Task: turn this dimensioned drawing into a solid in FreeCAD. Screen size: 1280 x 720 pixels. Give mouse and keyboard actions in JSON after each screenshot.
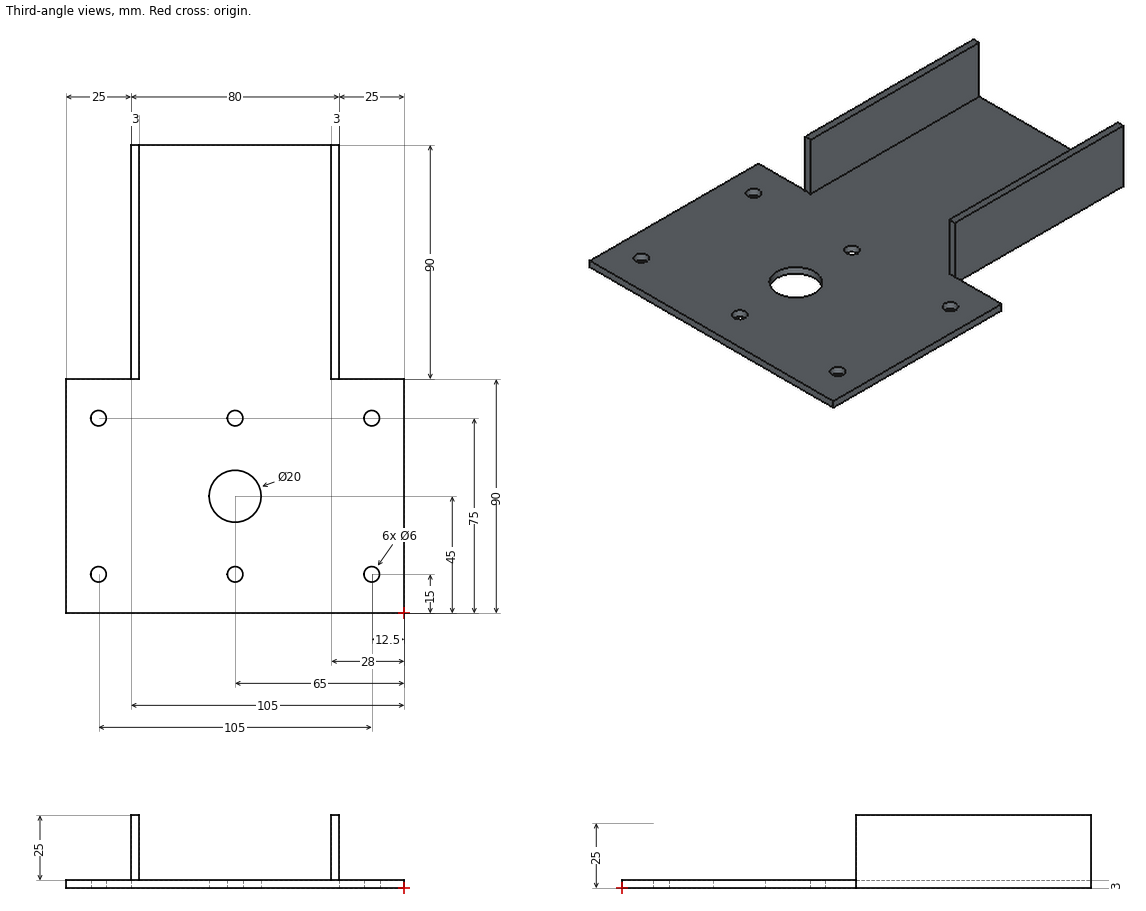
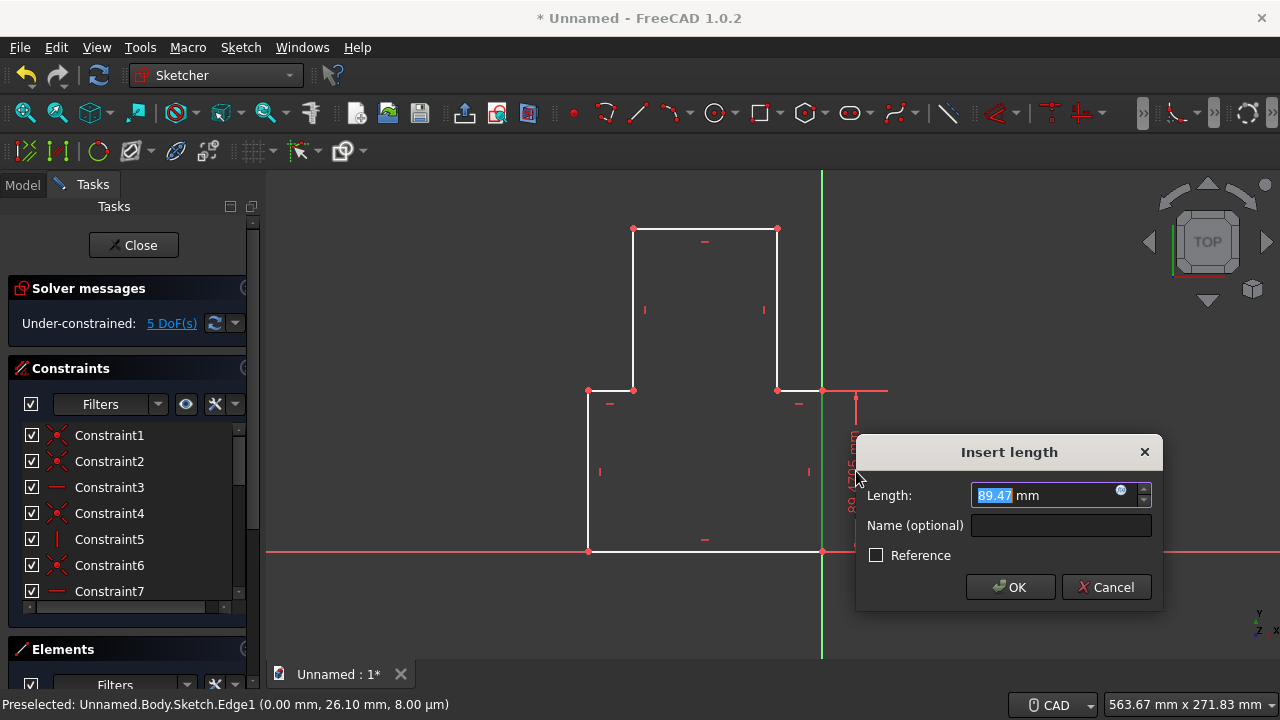
{"action": "type", "text": "90"}
{"action": "key", "text": "Return"}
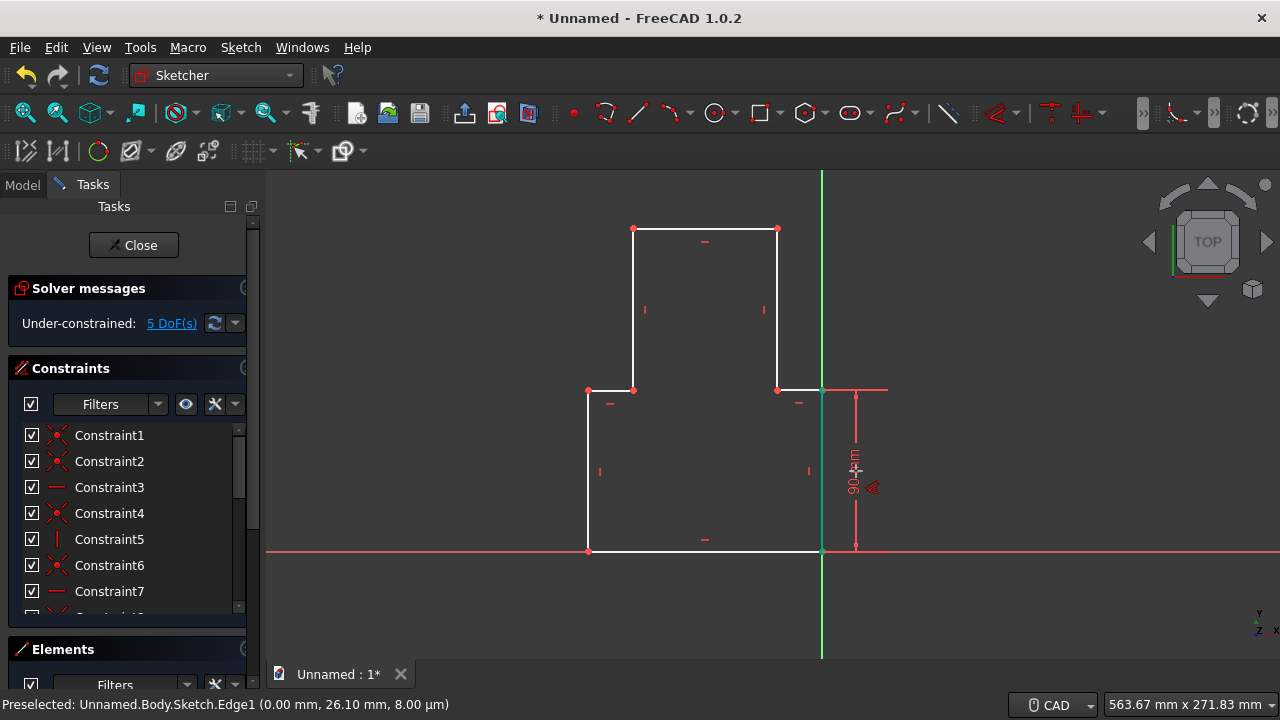
{"action": "left_click", "coordinate": [809, 390]}
{"action": "left_click", "coordinate": [800, 424]}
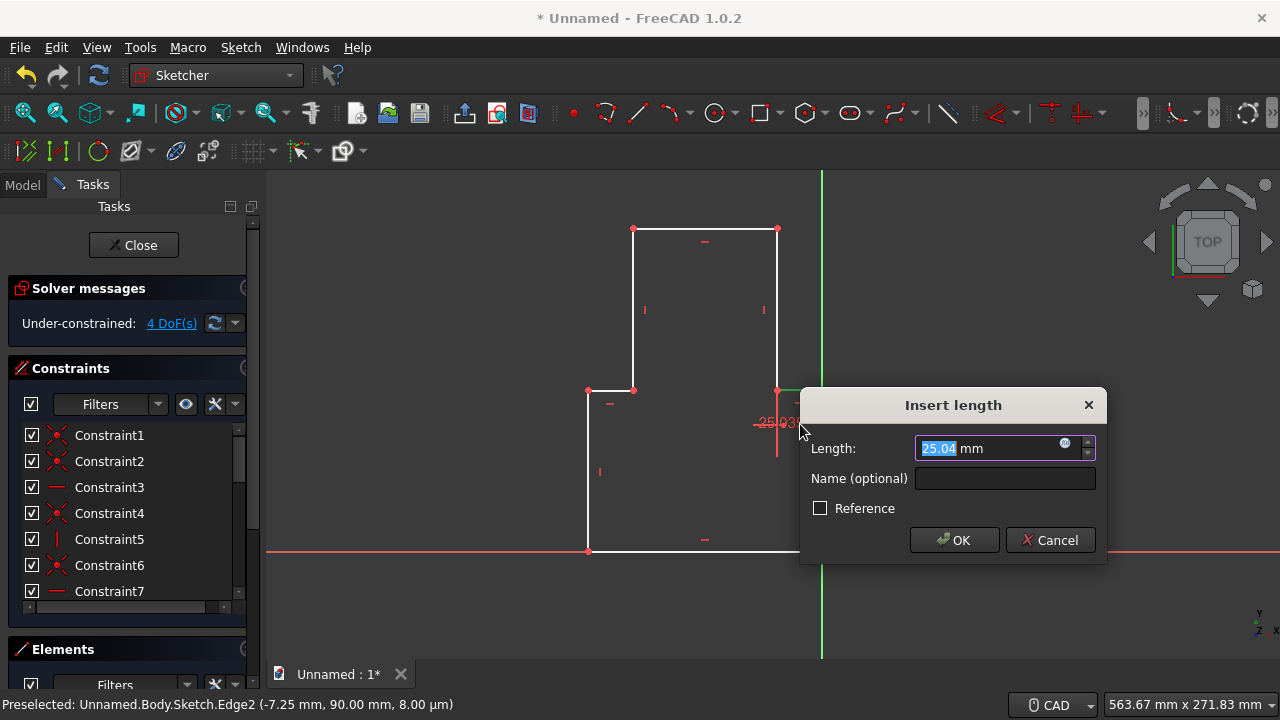
{"action": "type", "text": "25"}
{"action": "key", "text": "Return"}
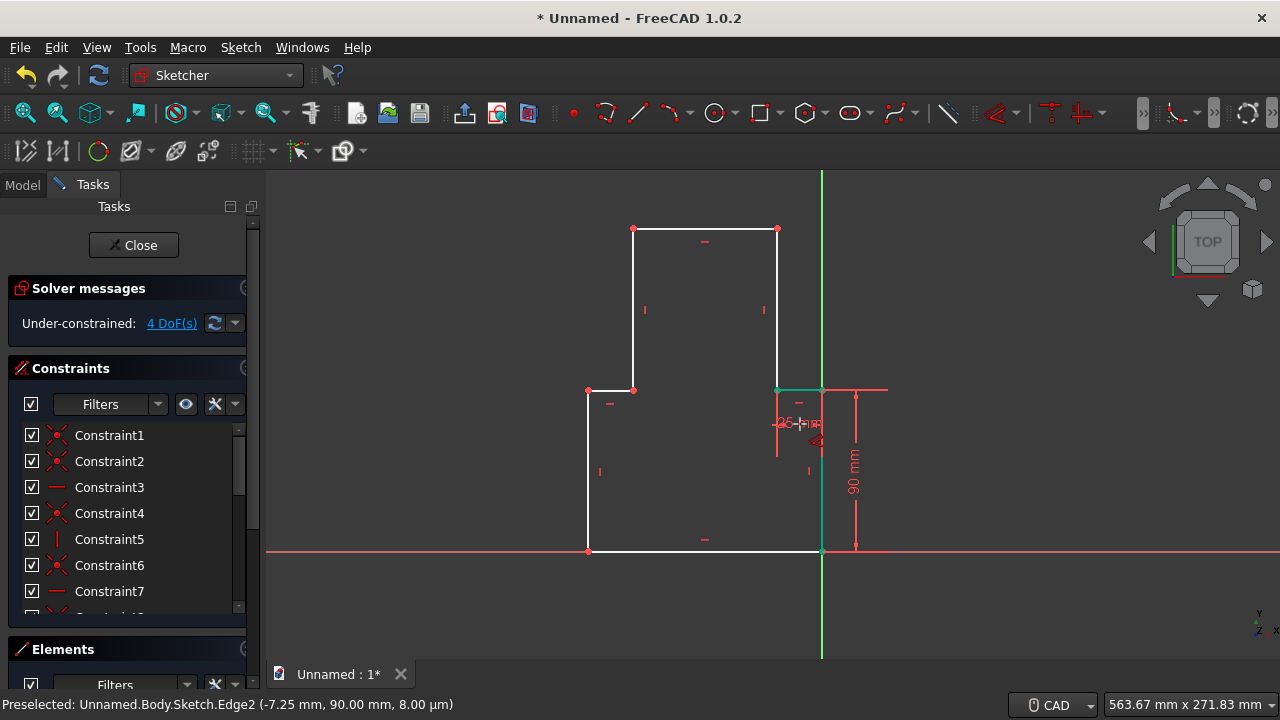
{"action": "left_click", "coordinate": [777, 342]}
{"action": "left_click", "coordinate": [743, 310]}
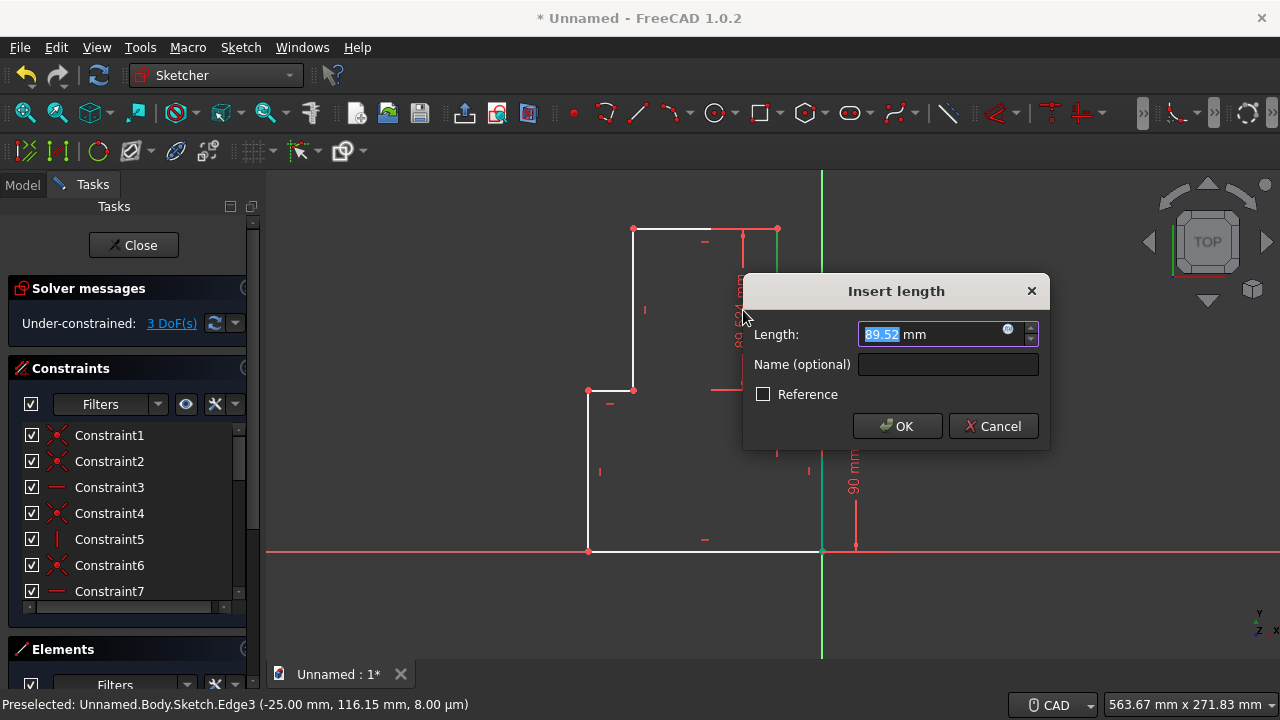
{"action": "type", "text": "90"}
{"action": "key", "text": "Return"}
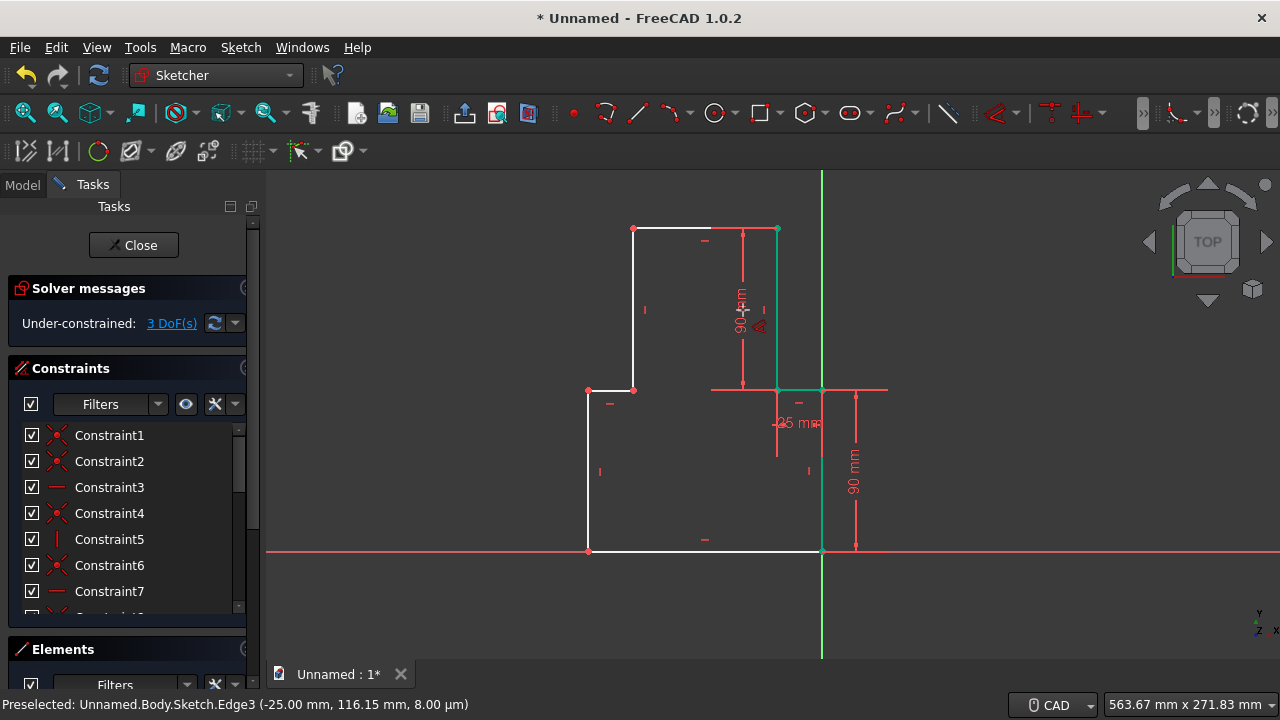
{"action": "left_click", "coordinate": [734, 228]}
{"action": "left_click", "coordinate": [705, 262]}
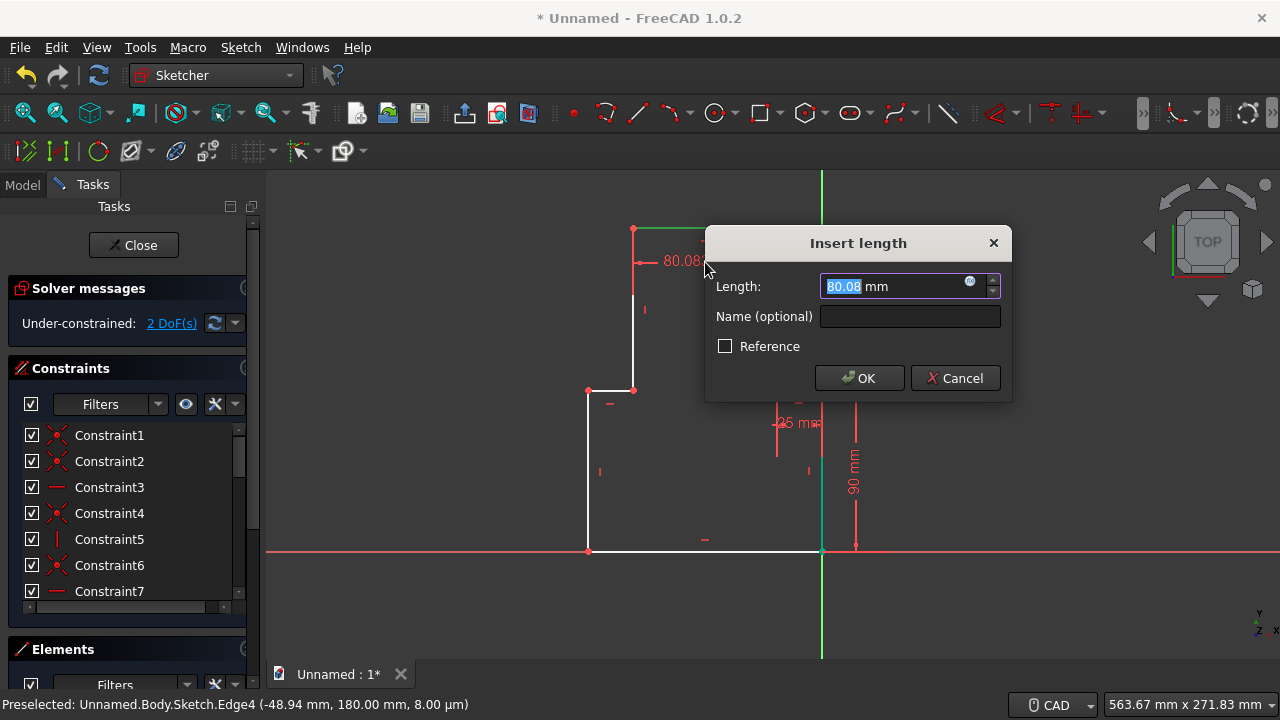
{"action": "type", "text": "80"}
{"action": "key", "text": "Return"}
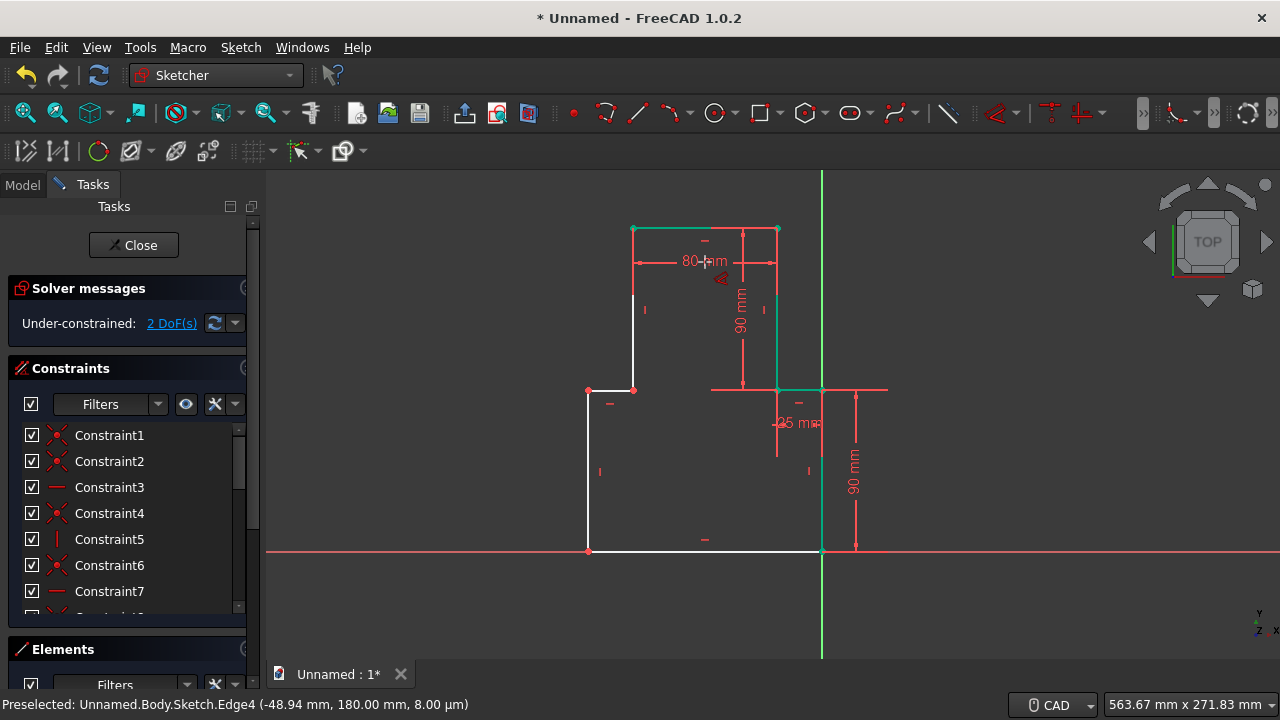
{"action": "left_click", "coordinate": [633, 277]}
{"action": "left_click", "coordinate": [599, 310]}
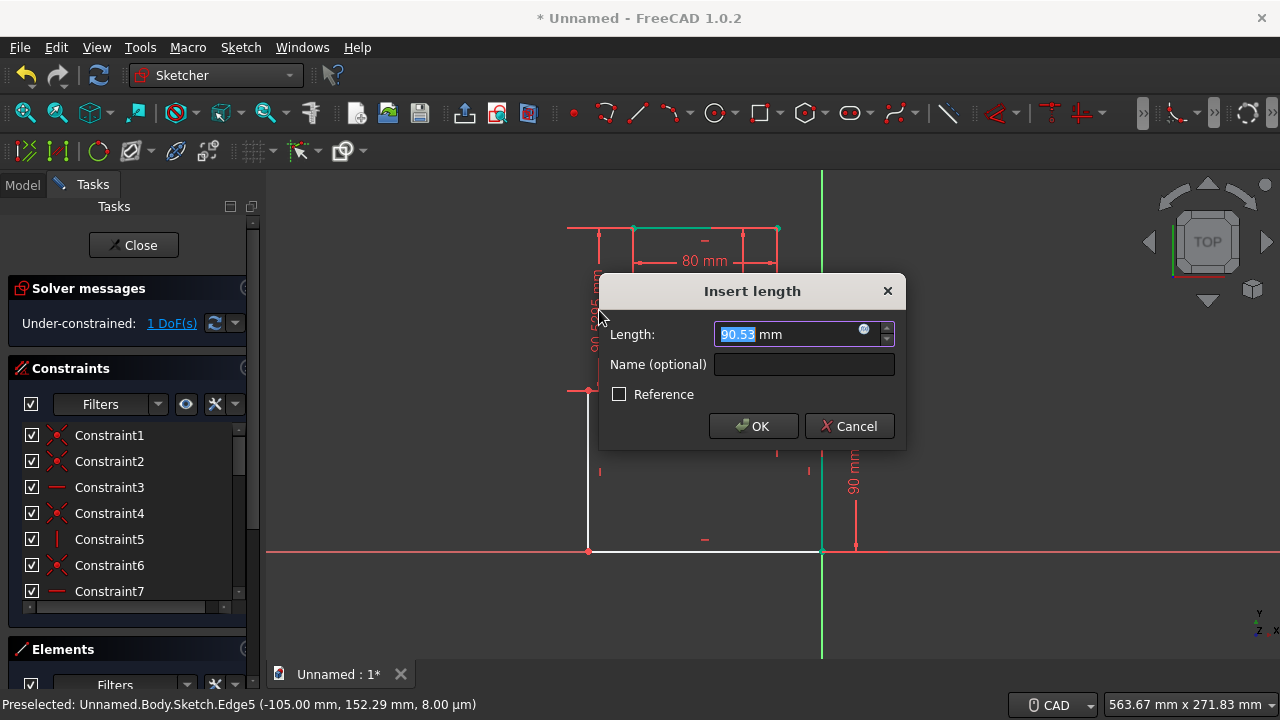
{"action": "type", "text": "90"}
{"action": "key", "text": "Return"}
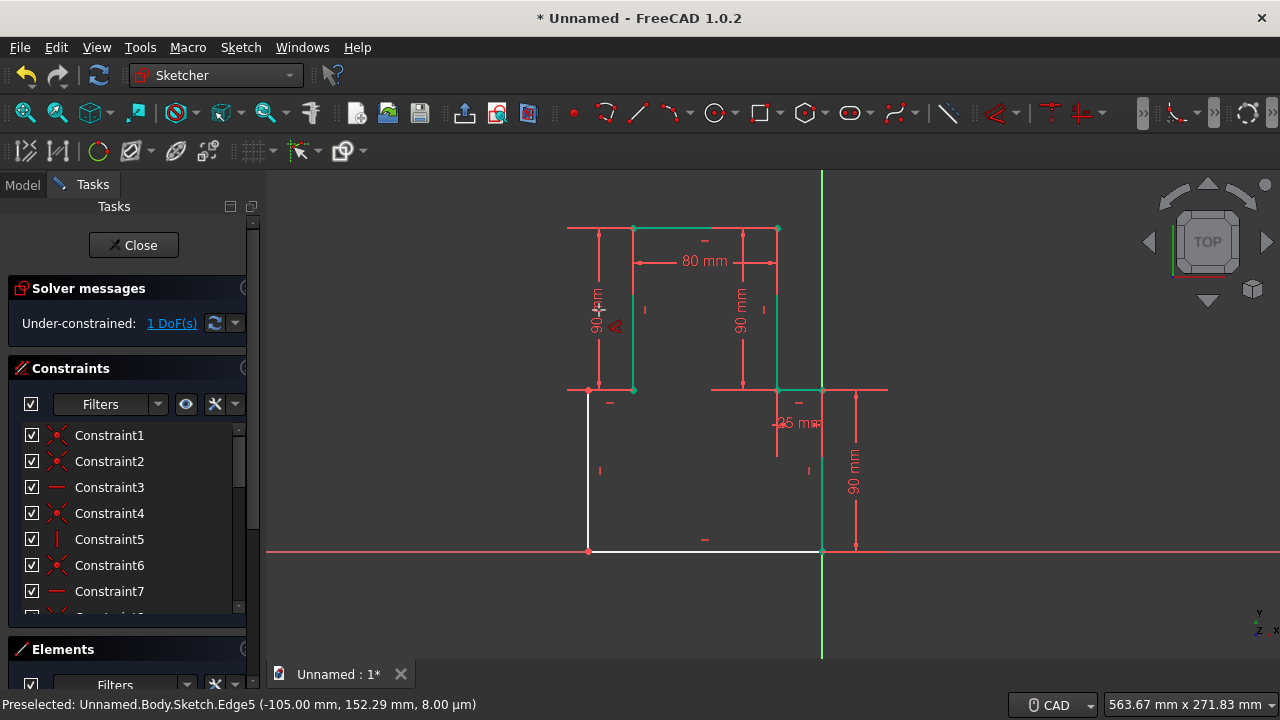
{"action": "left_click", "coordinate": [620, 390]}
{"action": "left_click", "coordinate": [611, 424]}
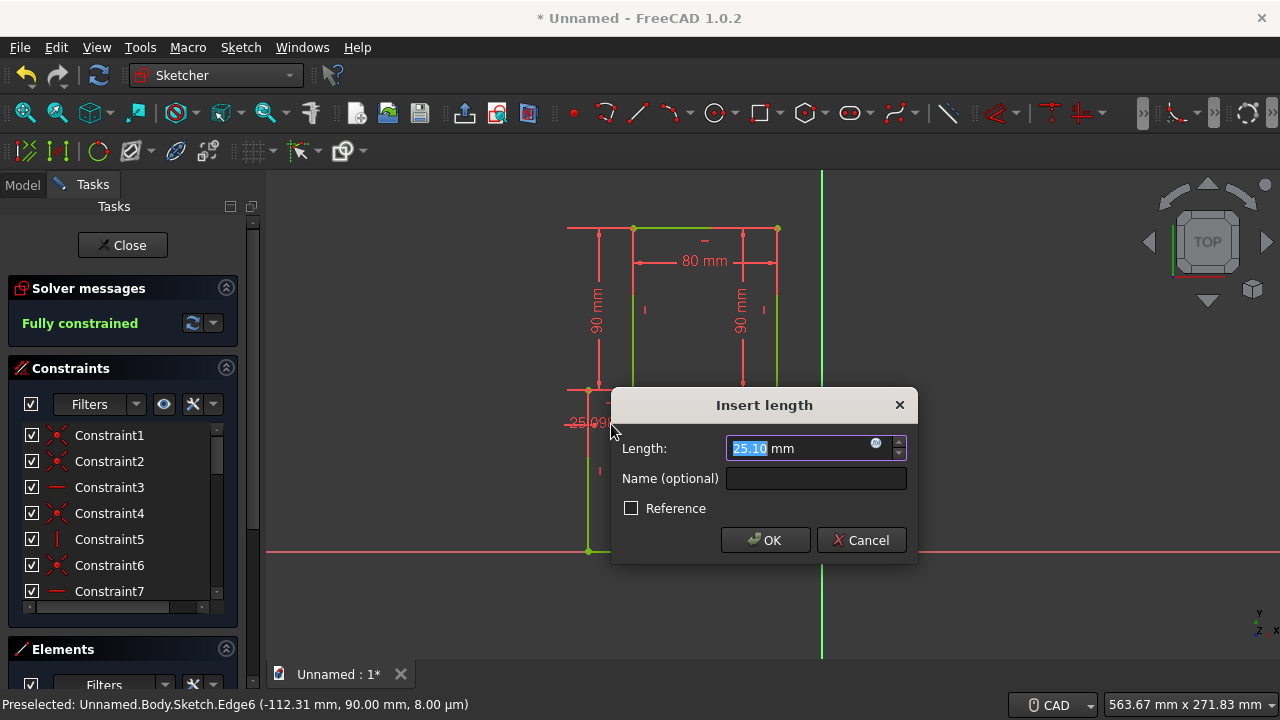
{"action": "type", "text": "25"}
{"action": "key", "text": "Return"}
{"action": "key", "text": "Escape"}